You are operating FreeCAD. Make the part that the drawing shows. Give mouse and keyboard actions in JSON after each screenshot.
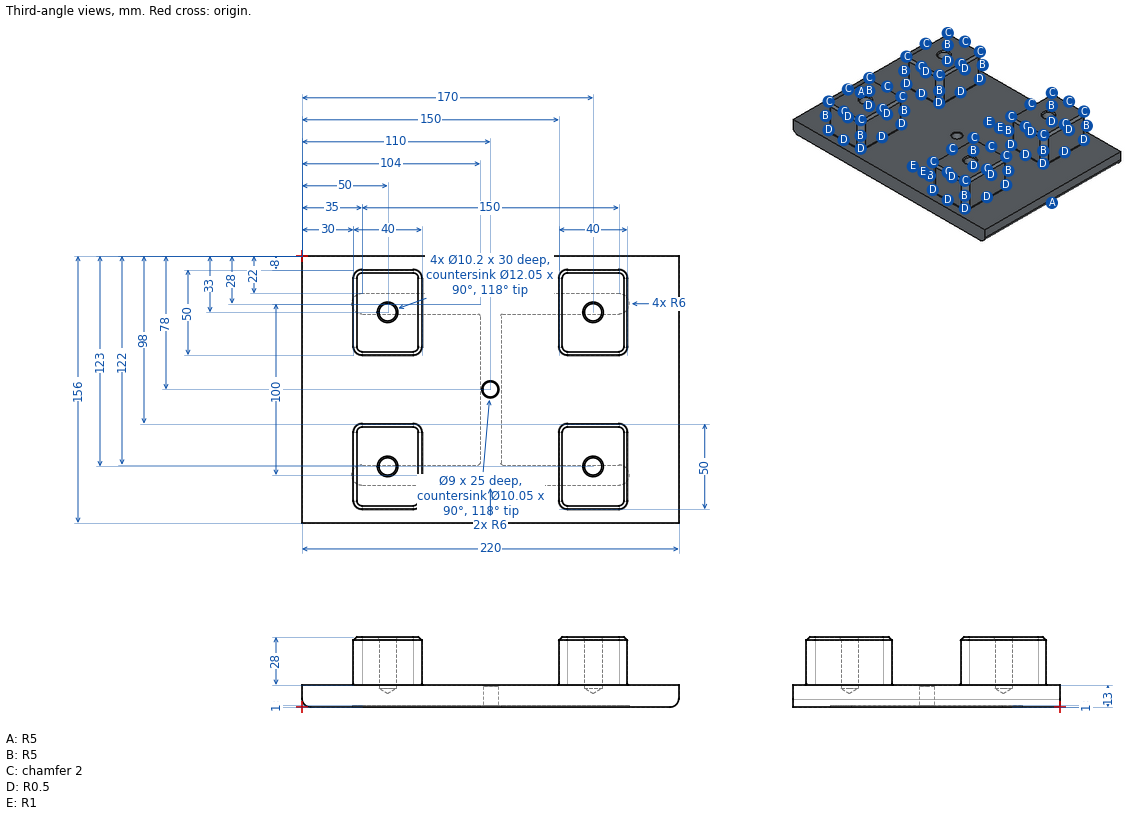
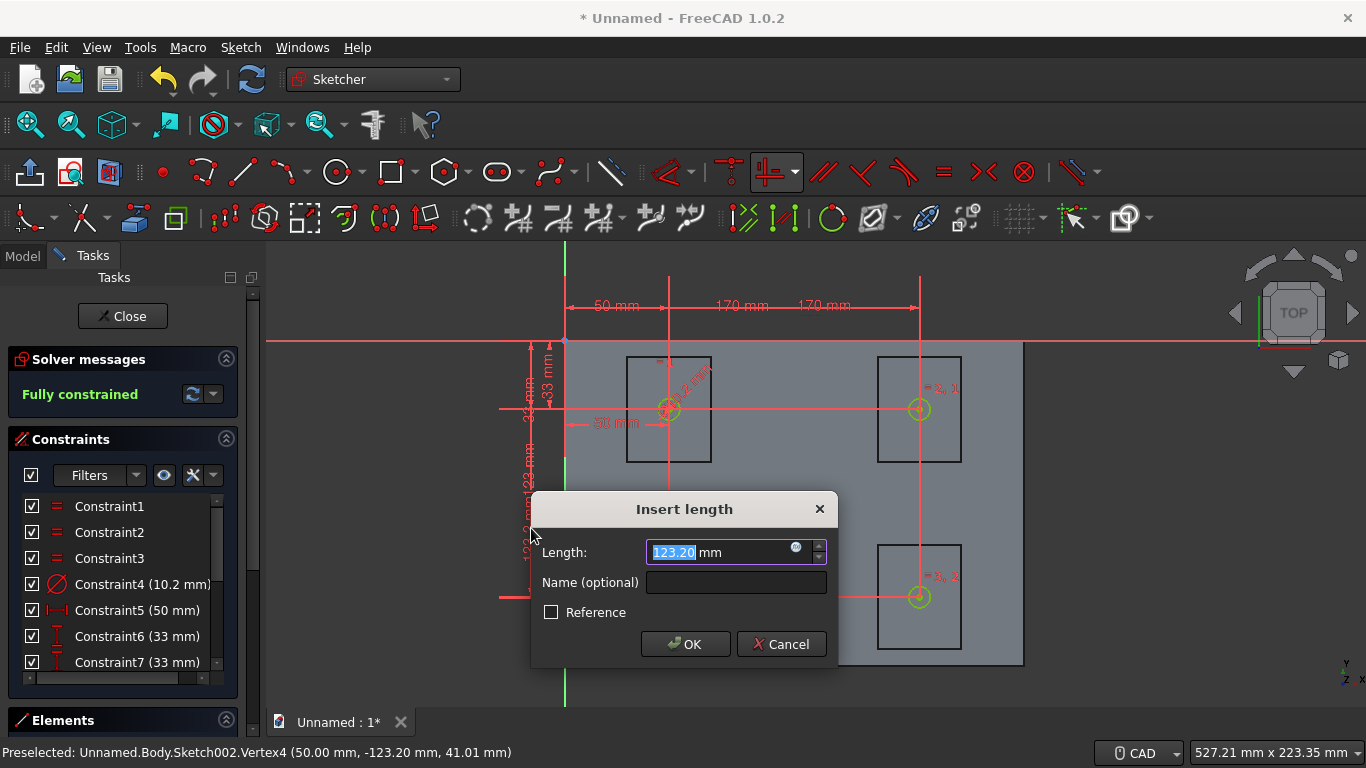
{"action": "type", "text": "123"}
{"action": "key", "text": "Return"}
{"action": "key", "text": "Escape"}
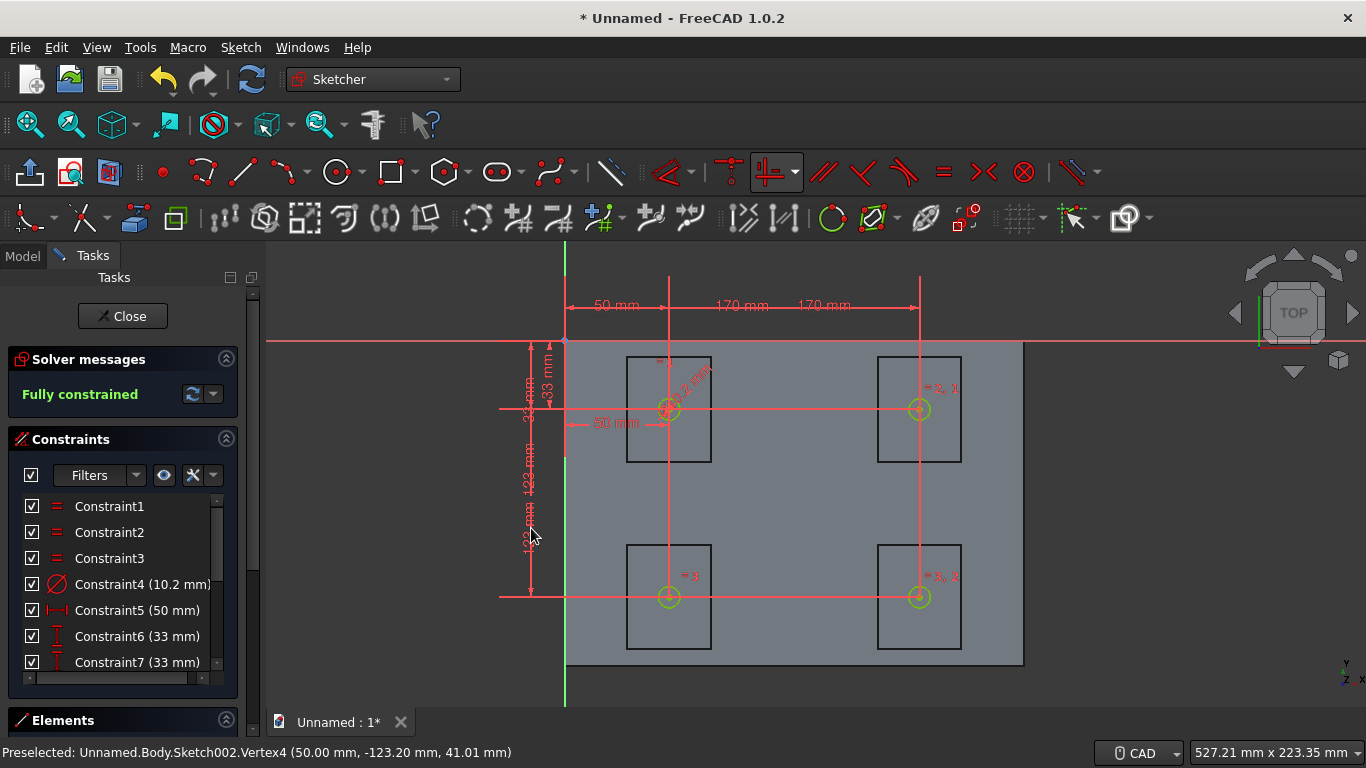
{"action": "left_click", "coordinate": [123, 316]}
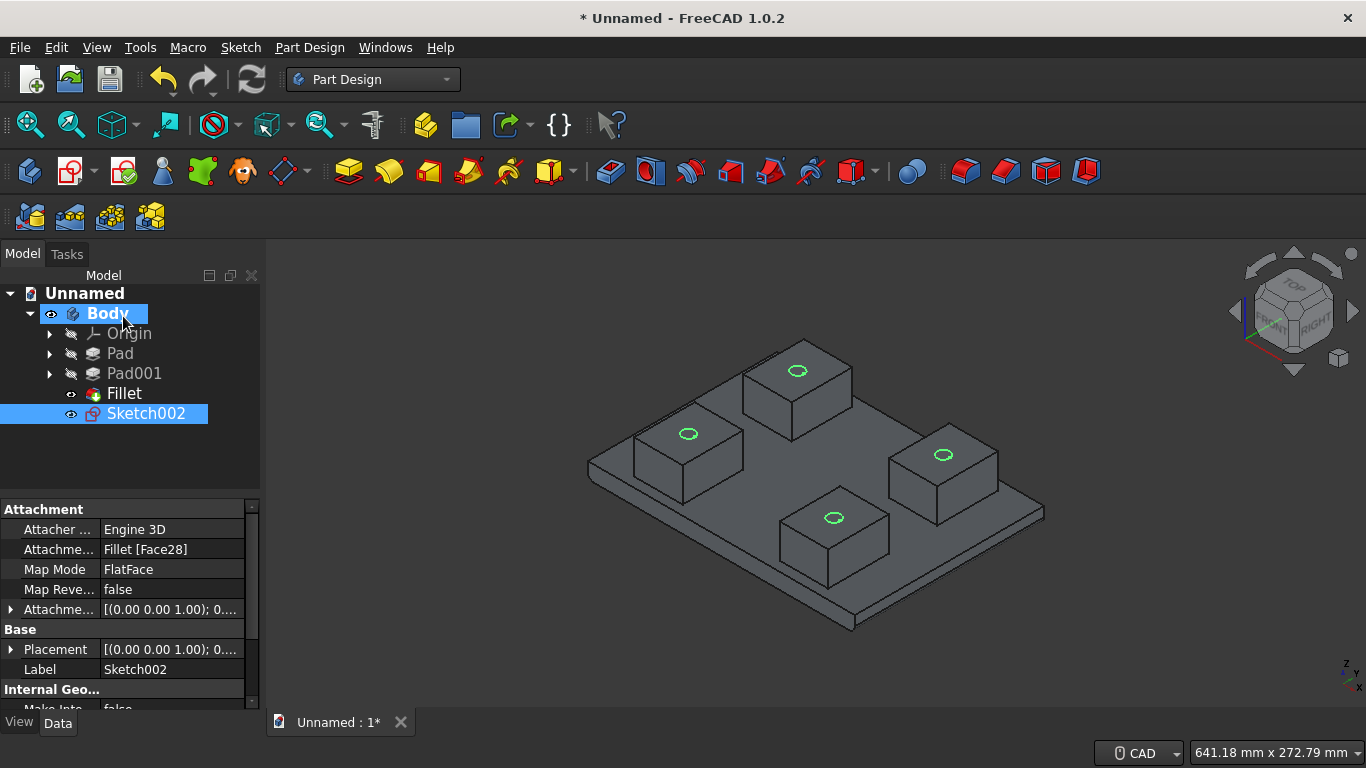
{"action": "left_click", "coordinate": [652, 172]}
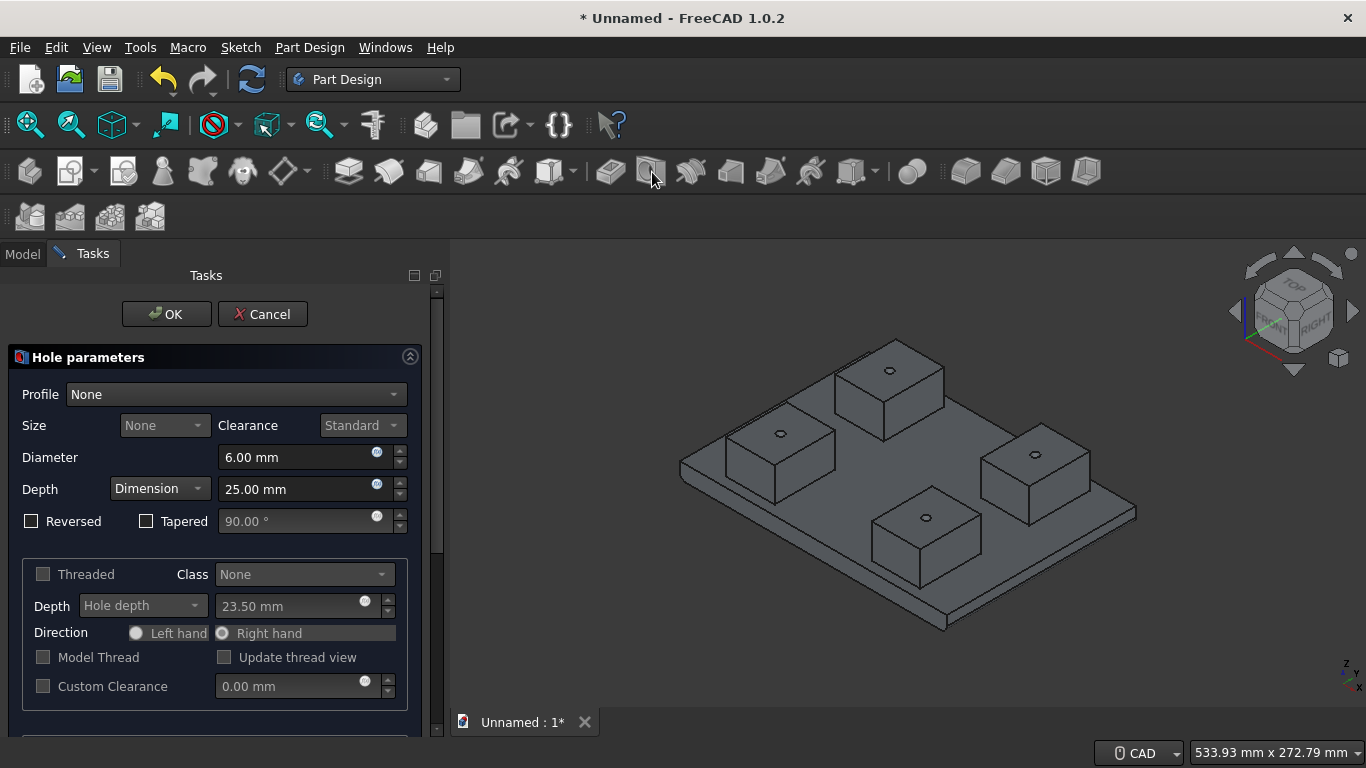
{"action": "triple_click", "coordinate": [305, 457]}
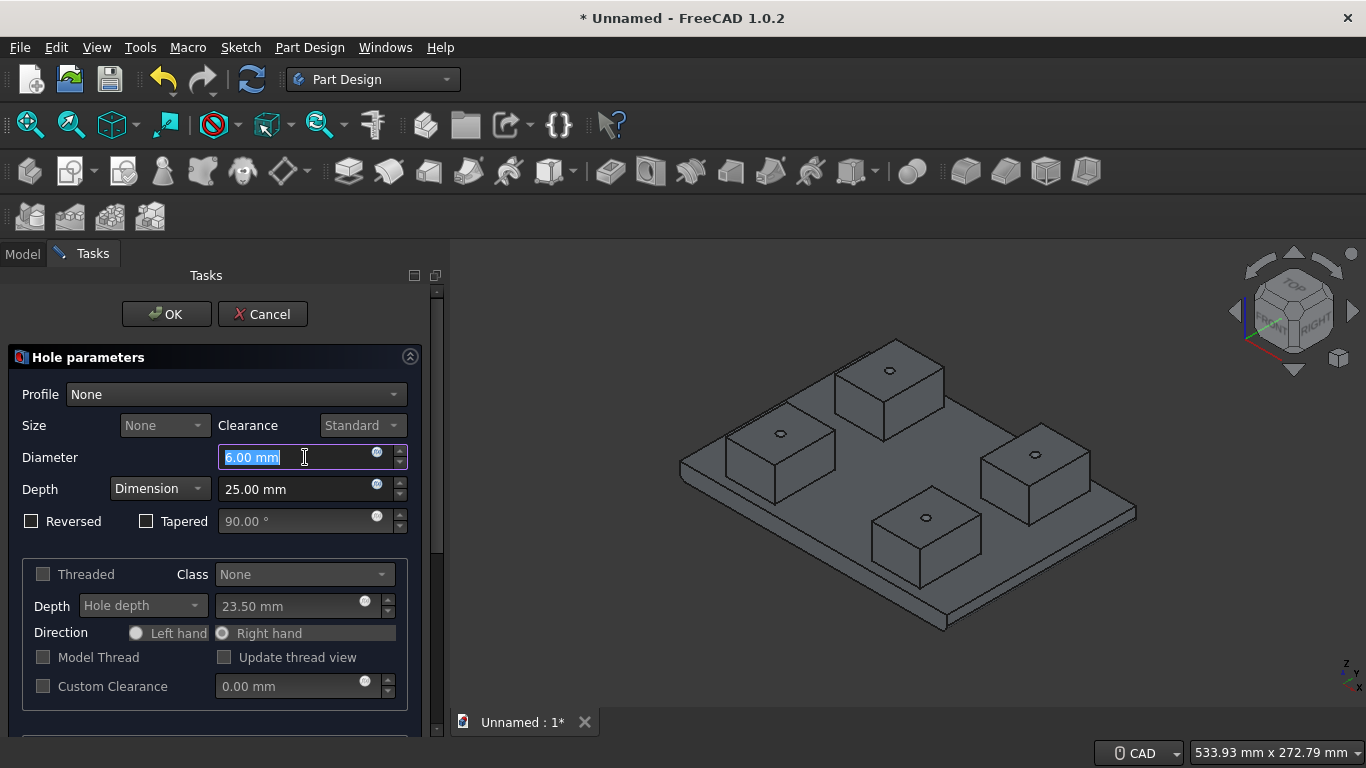
{"action": "type", "text": "10.2"}
{"action": "key", "text": "Tab"}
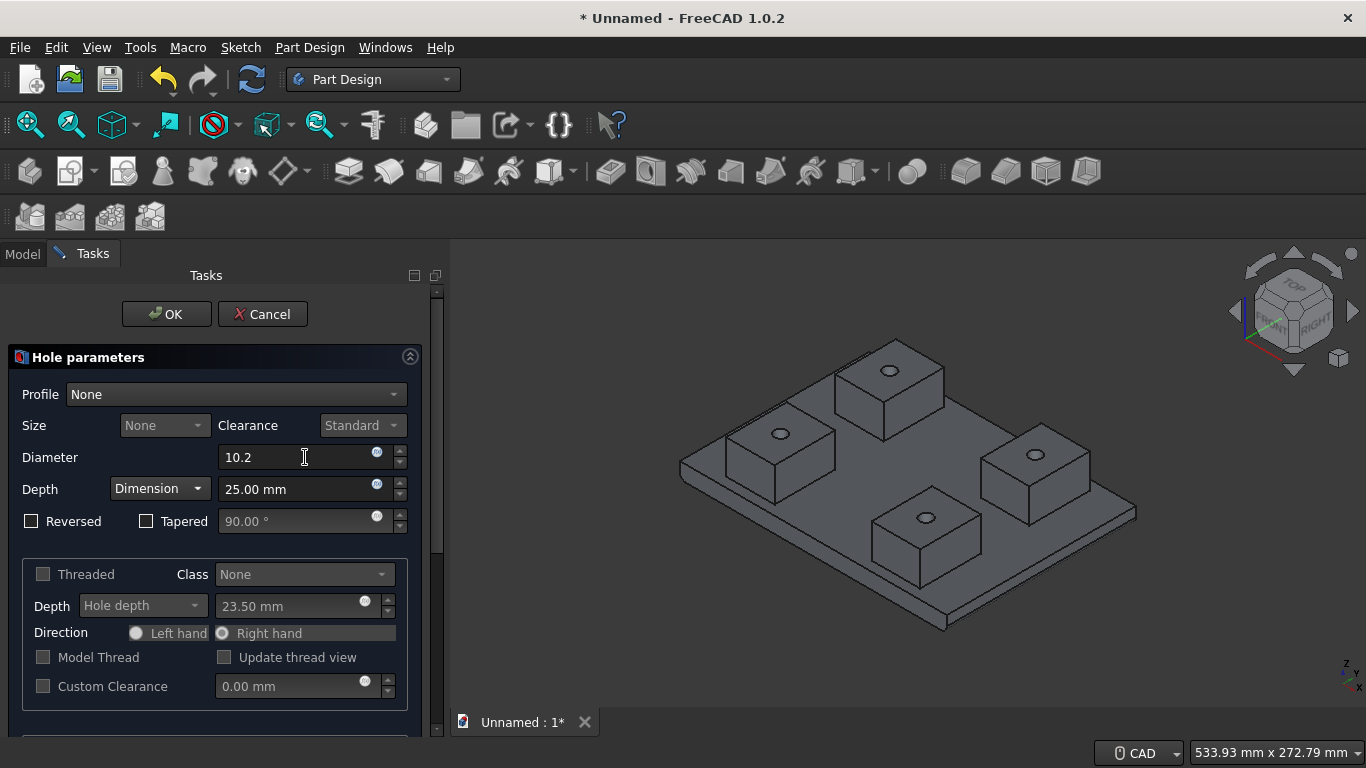
{"action": "triple_click", "coordinate": [305, 489]}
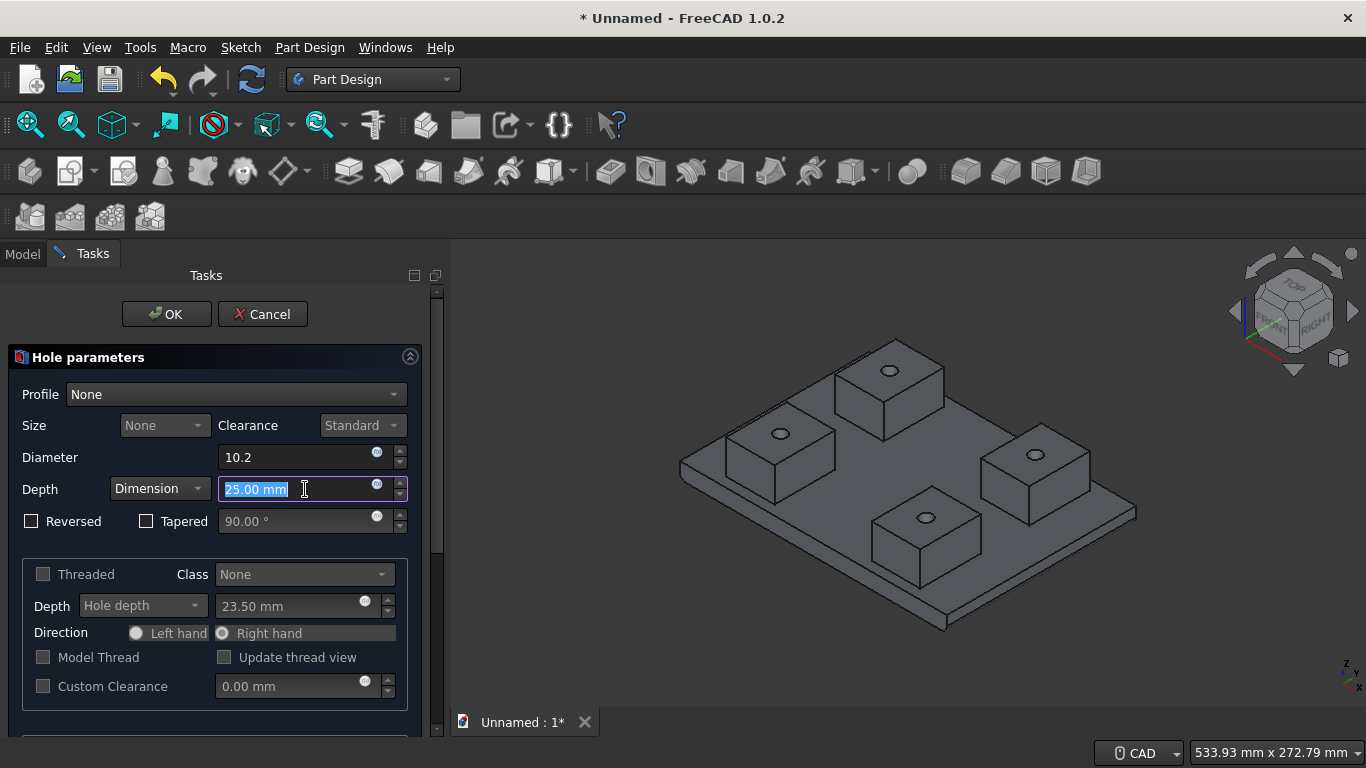
{"action": "type", "text": "30"}
{"action": "key", "text": "Tab"}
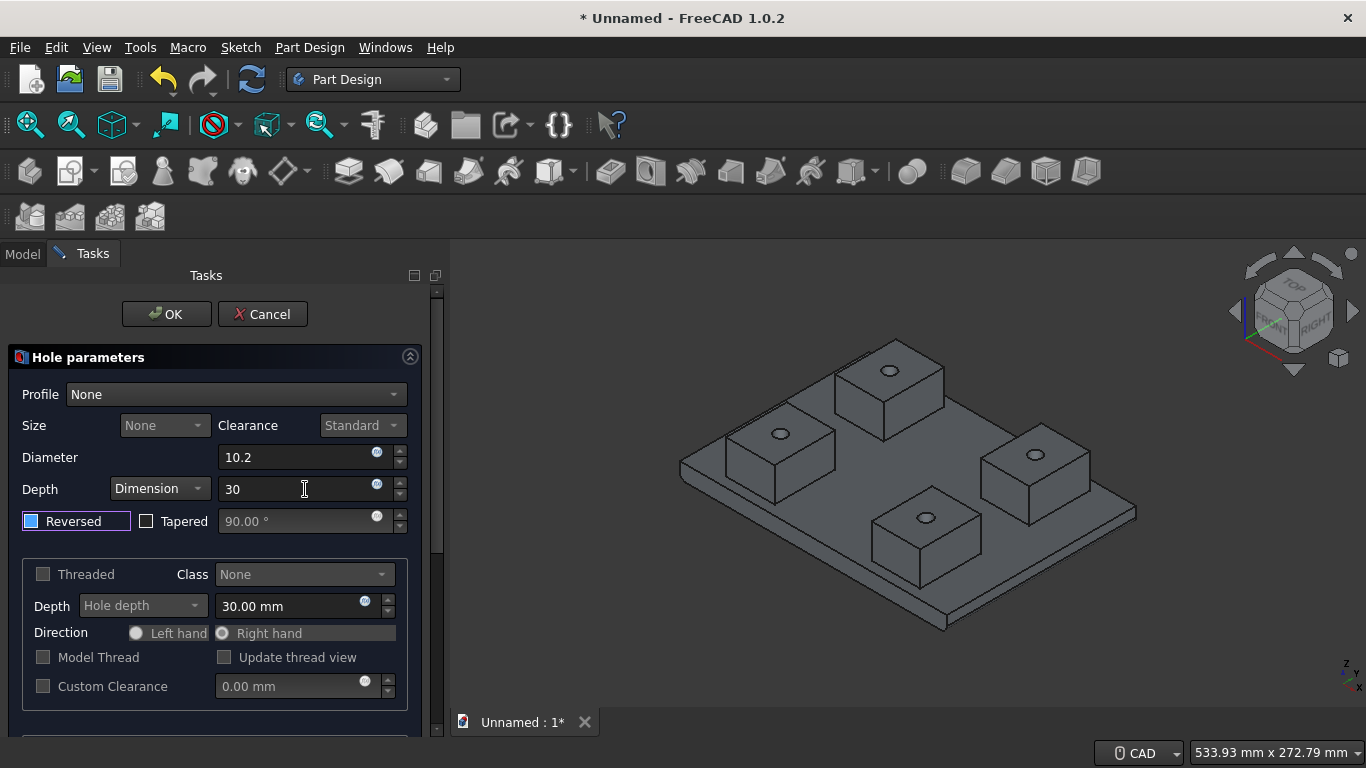
{"action": "scroll", "coordinate": [437, 510], "scroll_direction": "down", "scroll_amount": 2}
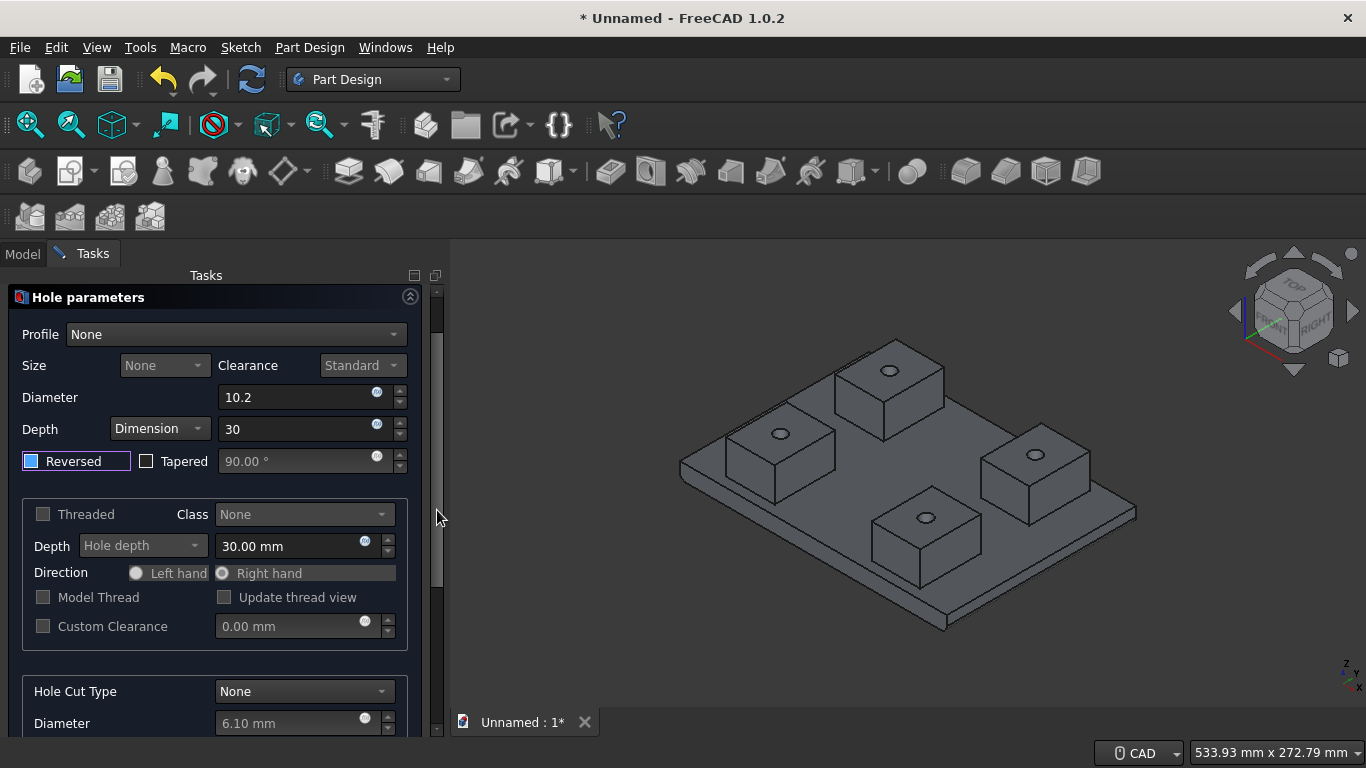
{"action": "left_click", "coordinate": [306, 632]}